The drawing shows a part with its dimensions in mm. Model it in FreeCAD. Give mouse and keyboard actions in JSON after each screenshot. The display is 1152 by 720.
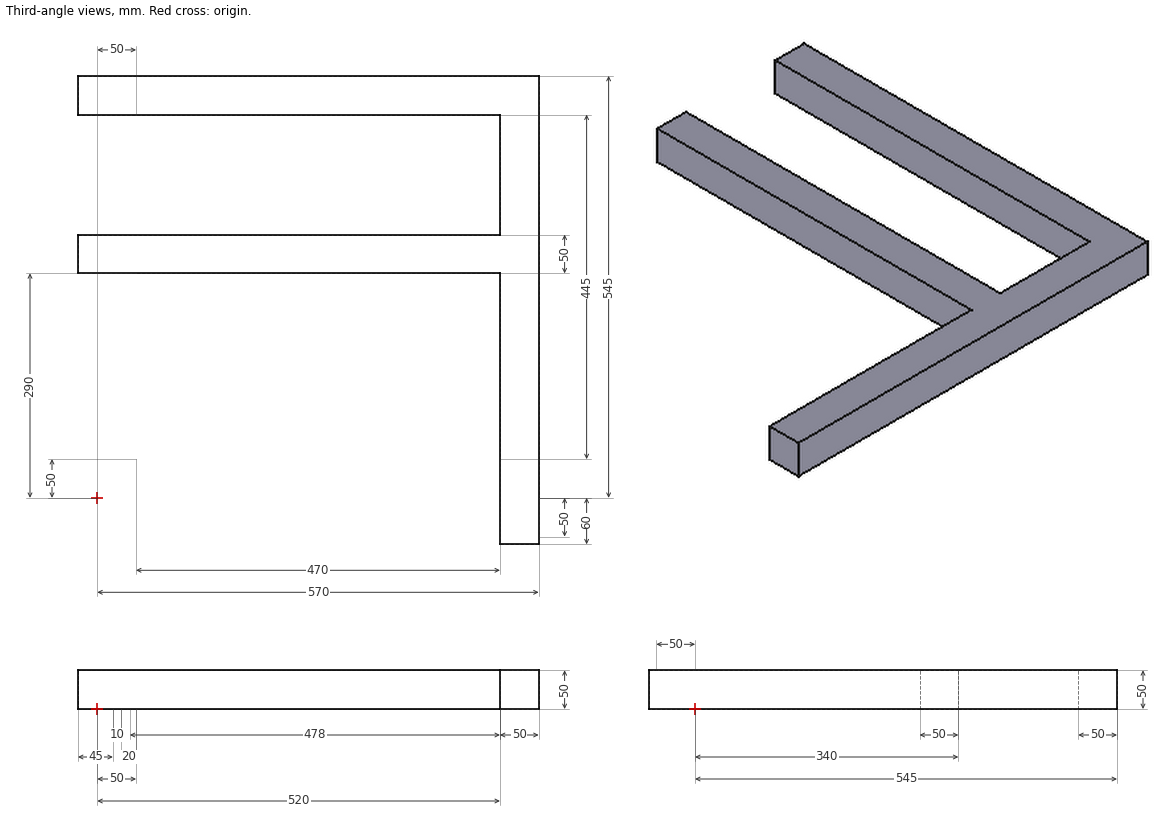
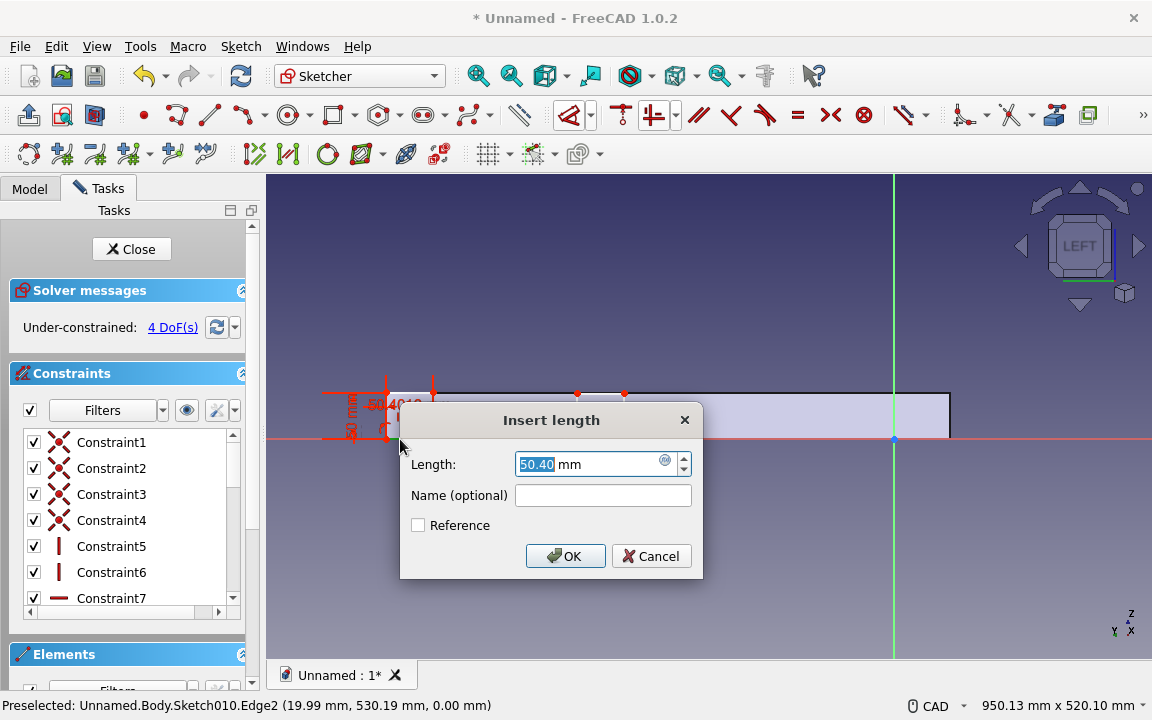
{"action": "type", "text": "50"}
{"action": "key", "text": "Return"}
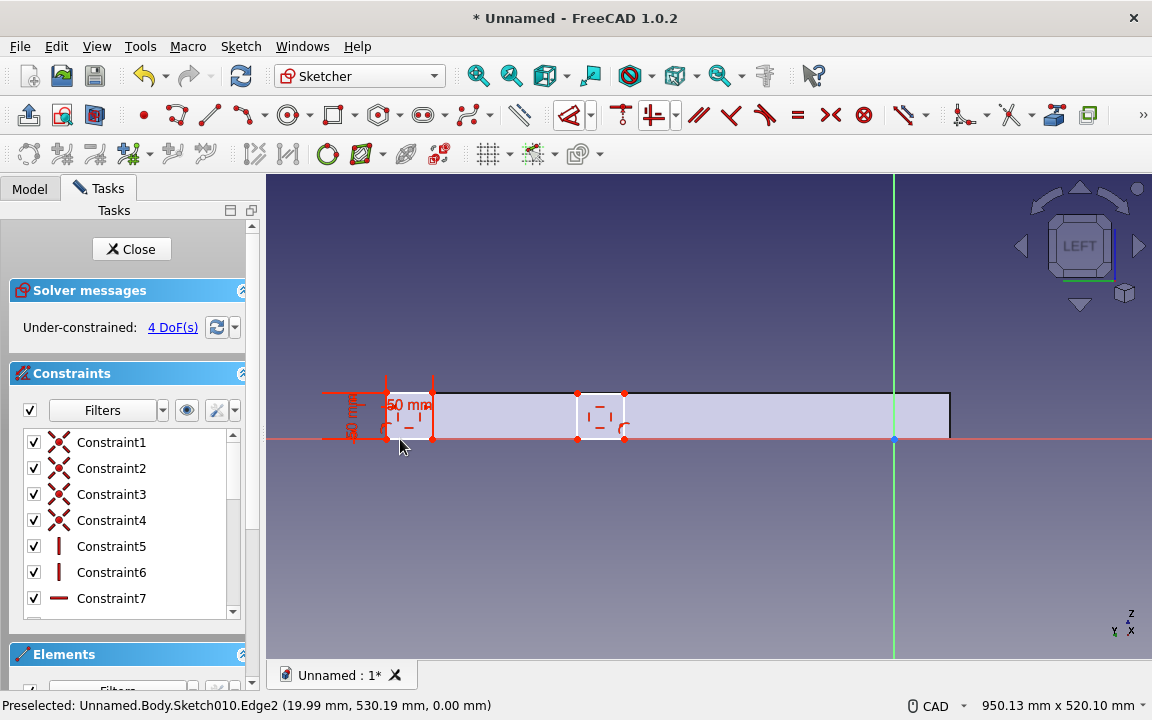
{"action": "left_click", "coordinate": [577, 408]}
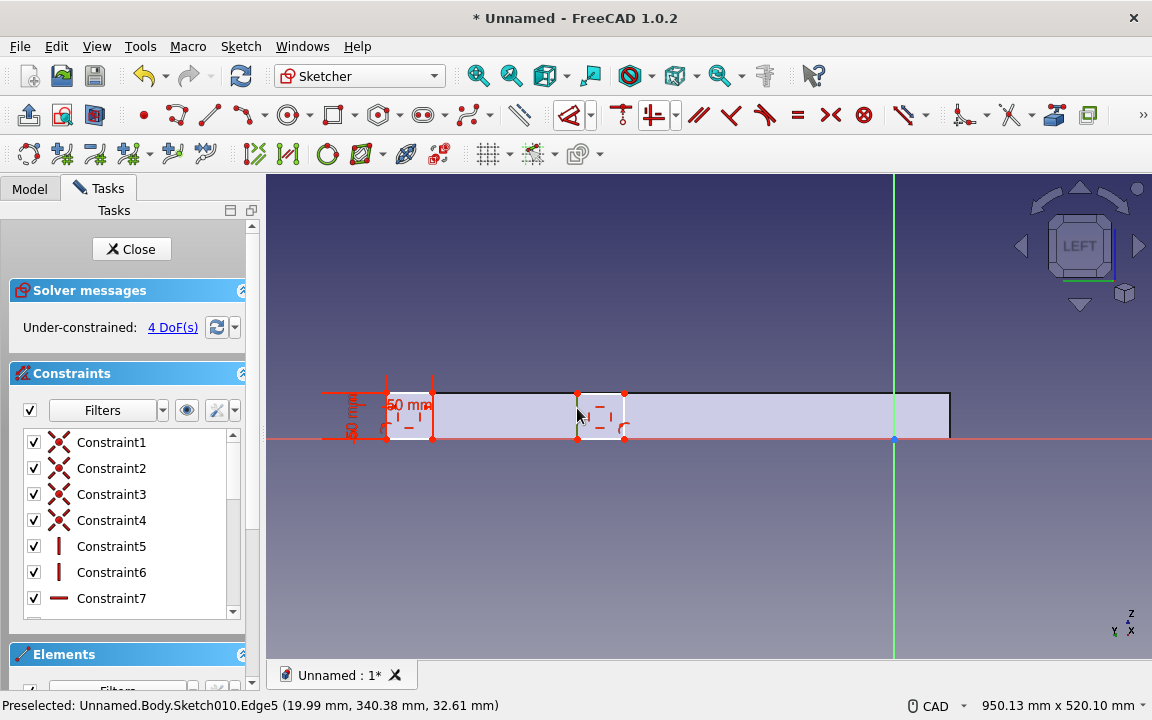
{"action": "key", "text": "i"}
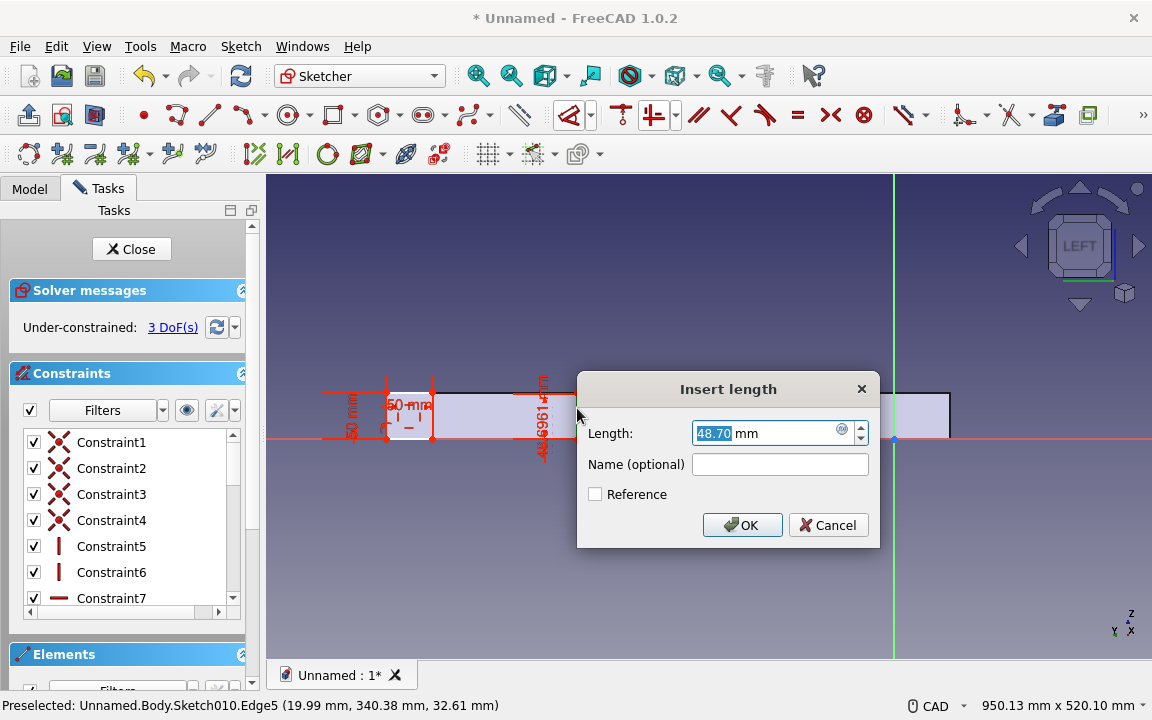
{"action": "type", "text": "50"}
{"action": "key", "text": "Return"}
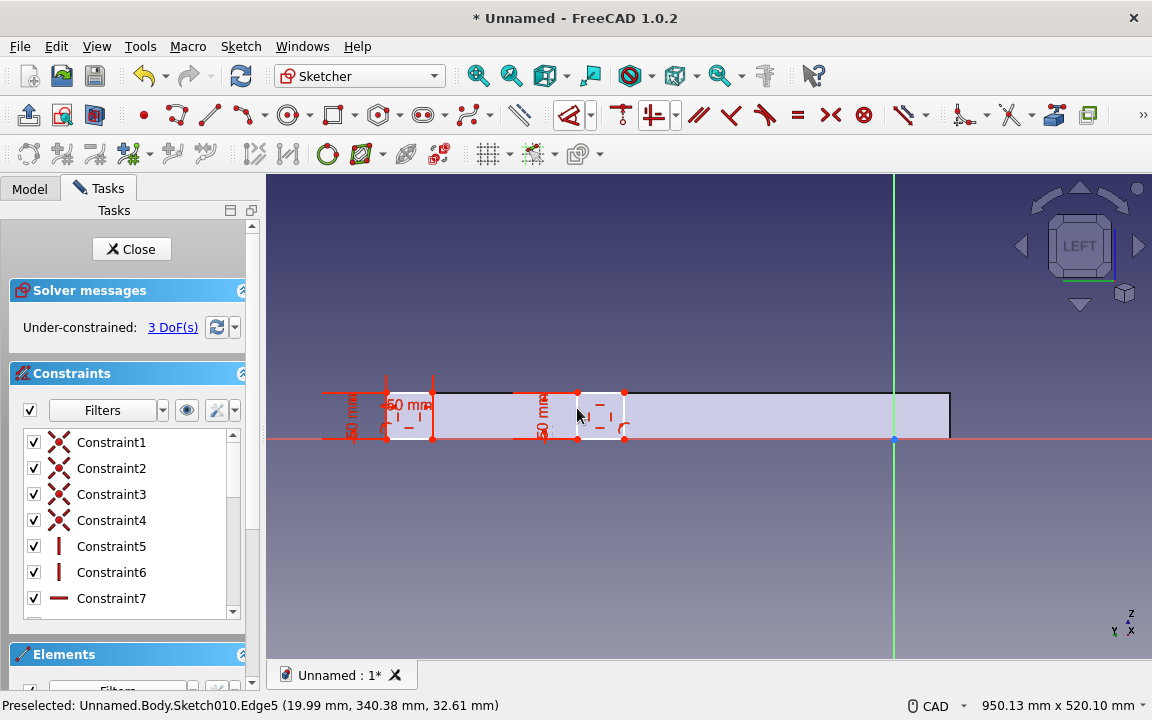
{"action": "left_click", "coordinate": [591, 439]}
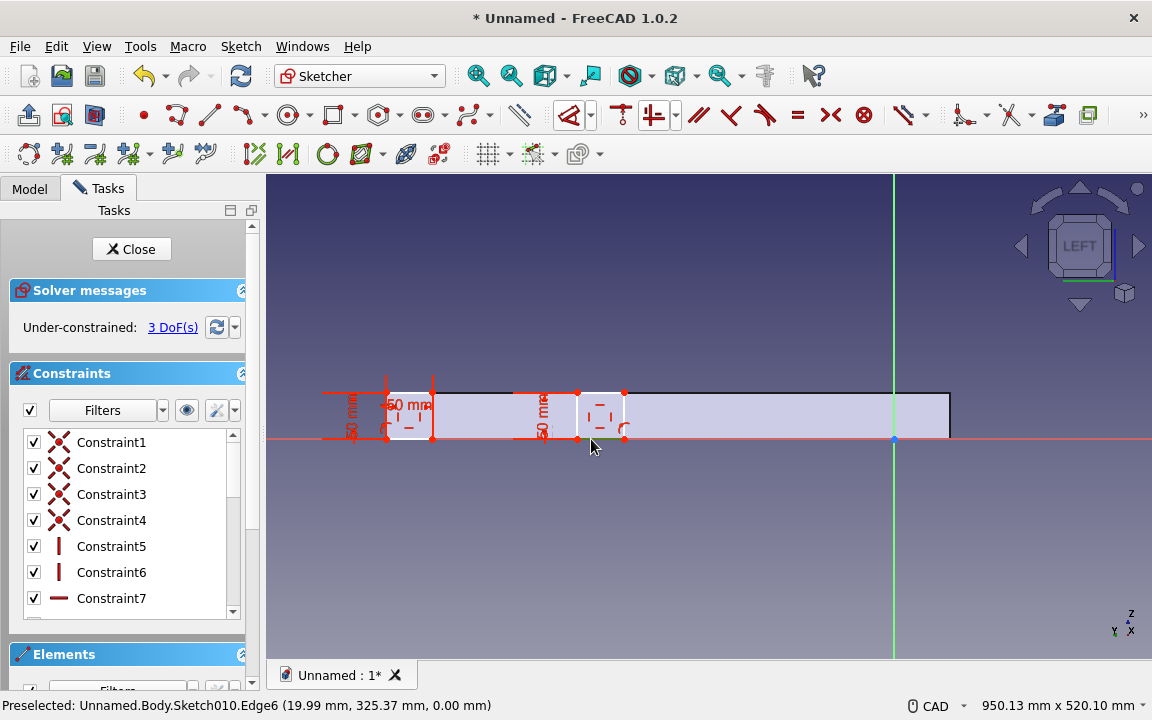
{"action": "key", "text": "l"}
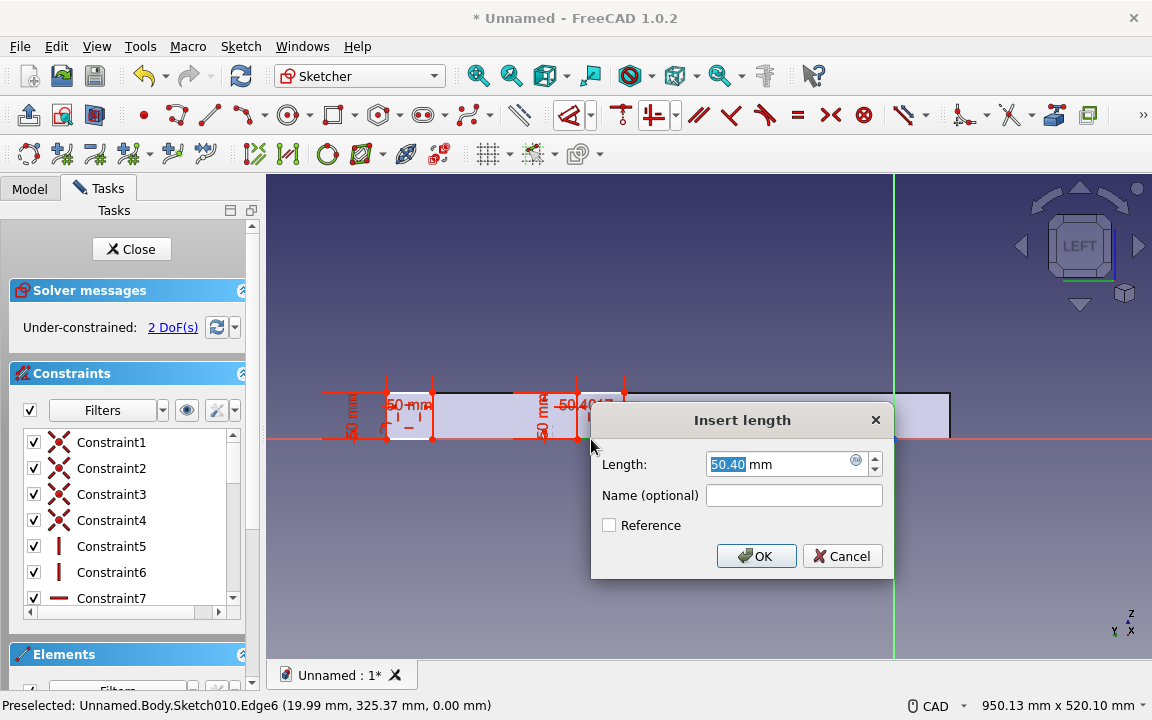
{"action": "type", "text": "50"}
{"action": "key", "text": "Return"}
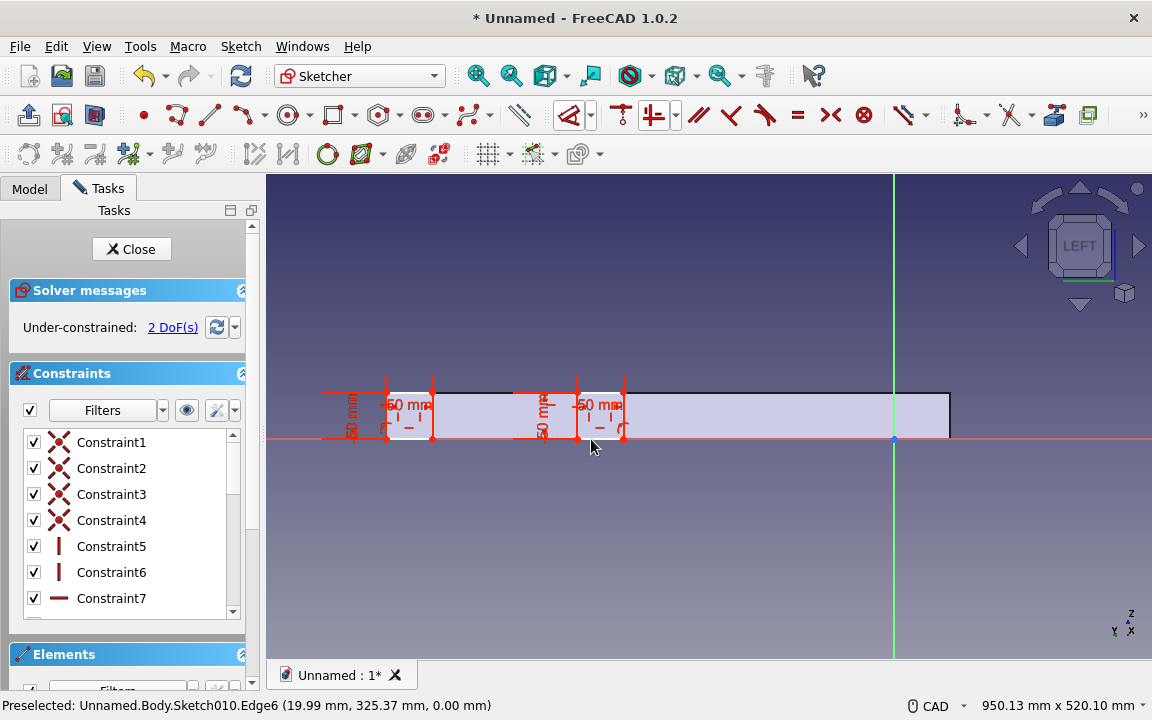
{"action": "left_click", "coordinate": [386, 393]}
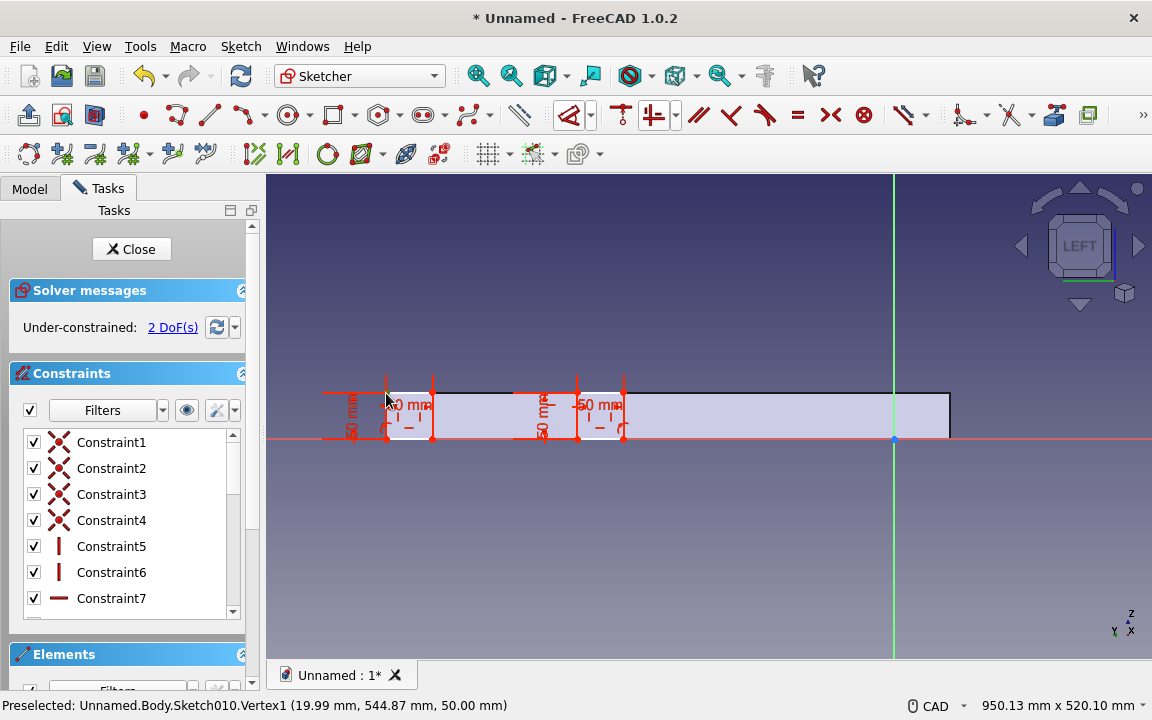
{"action": "key", "text": "l"}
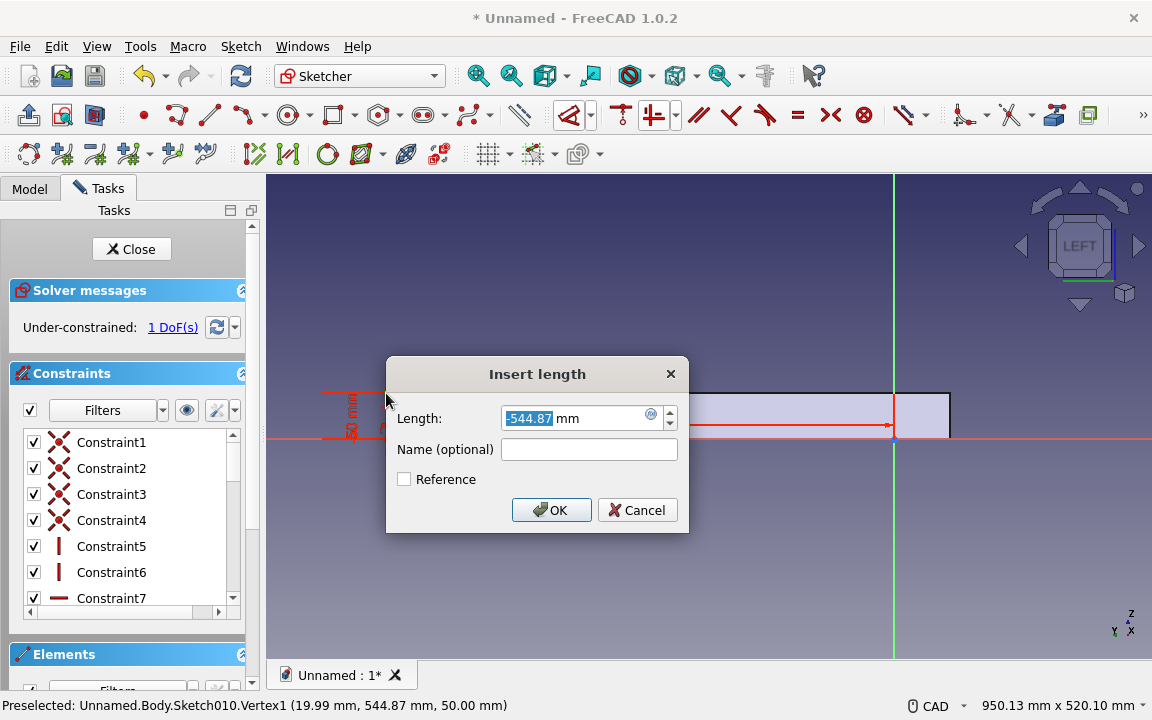
{"action": "type", "text": "-545"}
{"action": "key", "text": "Return"}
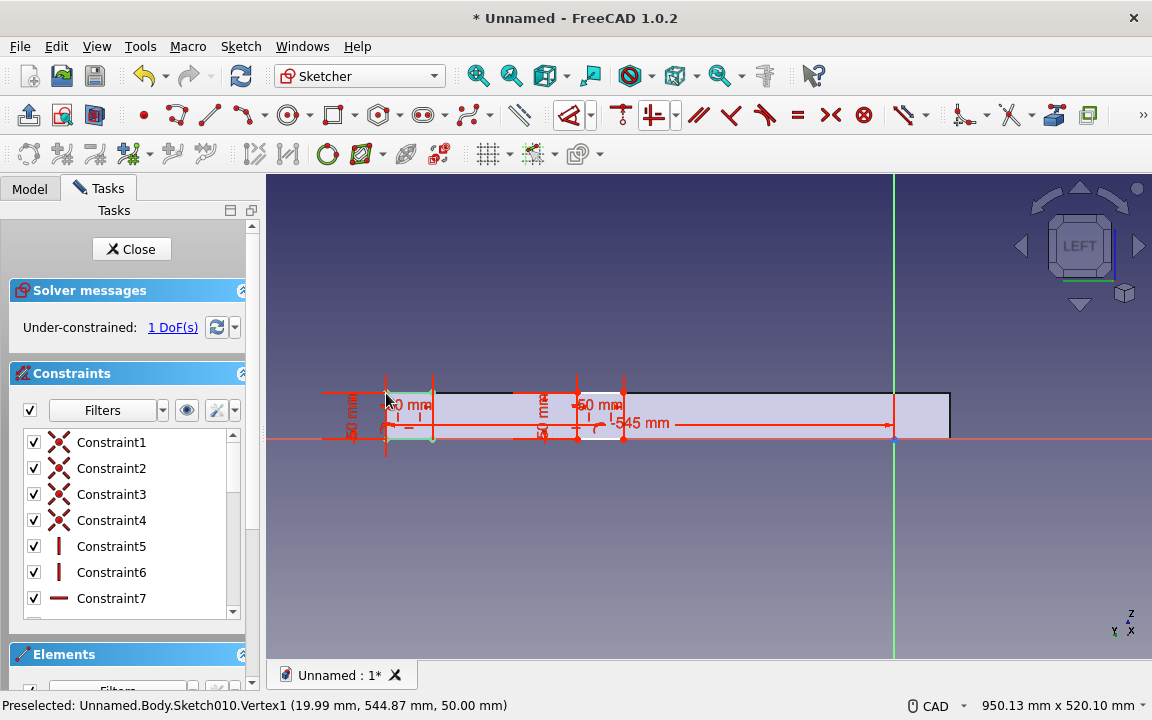
{"action": "left_click", "coordinate": [577, 393]}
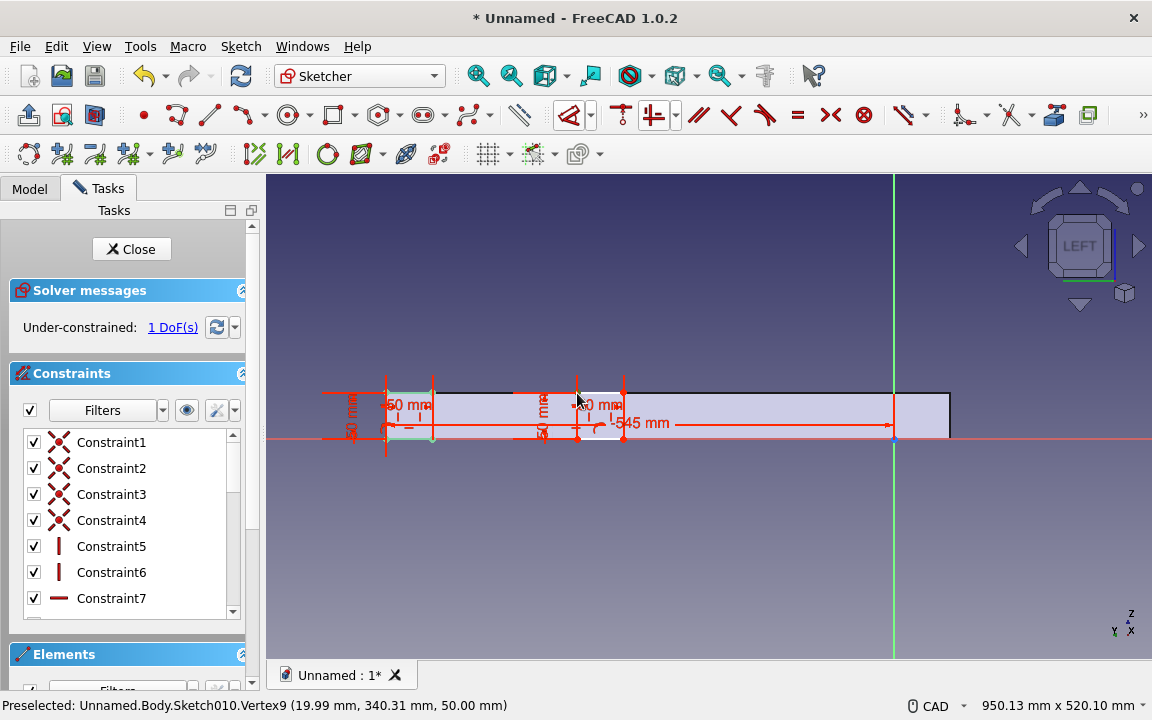
{"action": "left_click", "coordinate": [590, 116]}